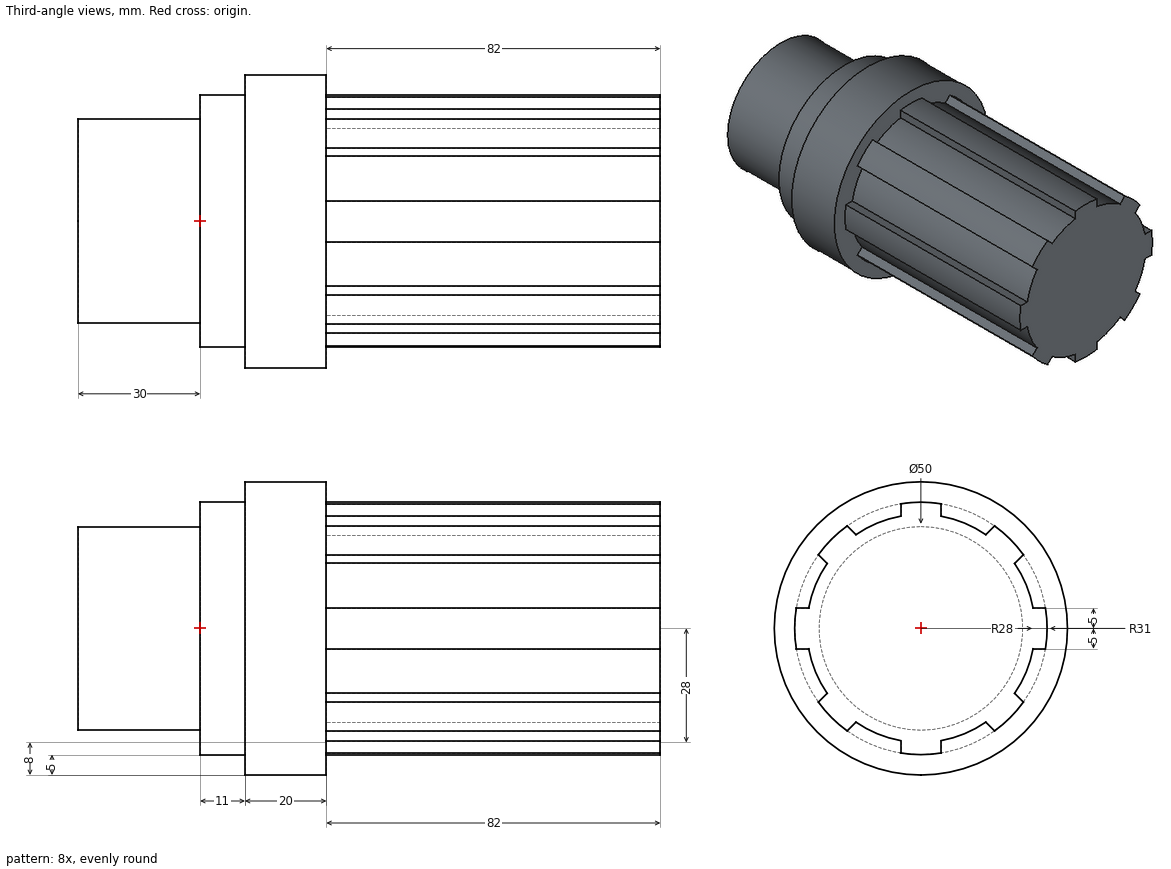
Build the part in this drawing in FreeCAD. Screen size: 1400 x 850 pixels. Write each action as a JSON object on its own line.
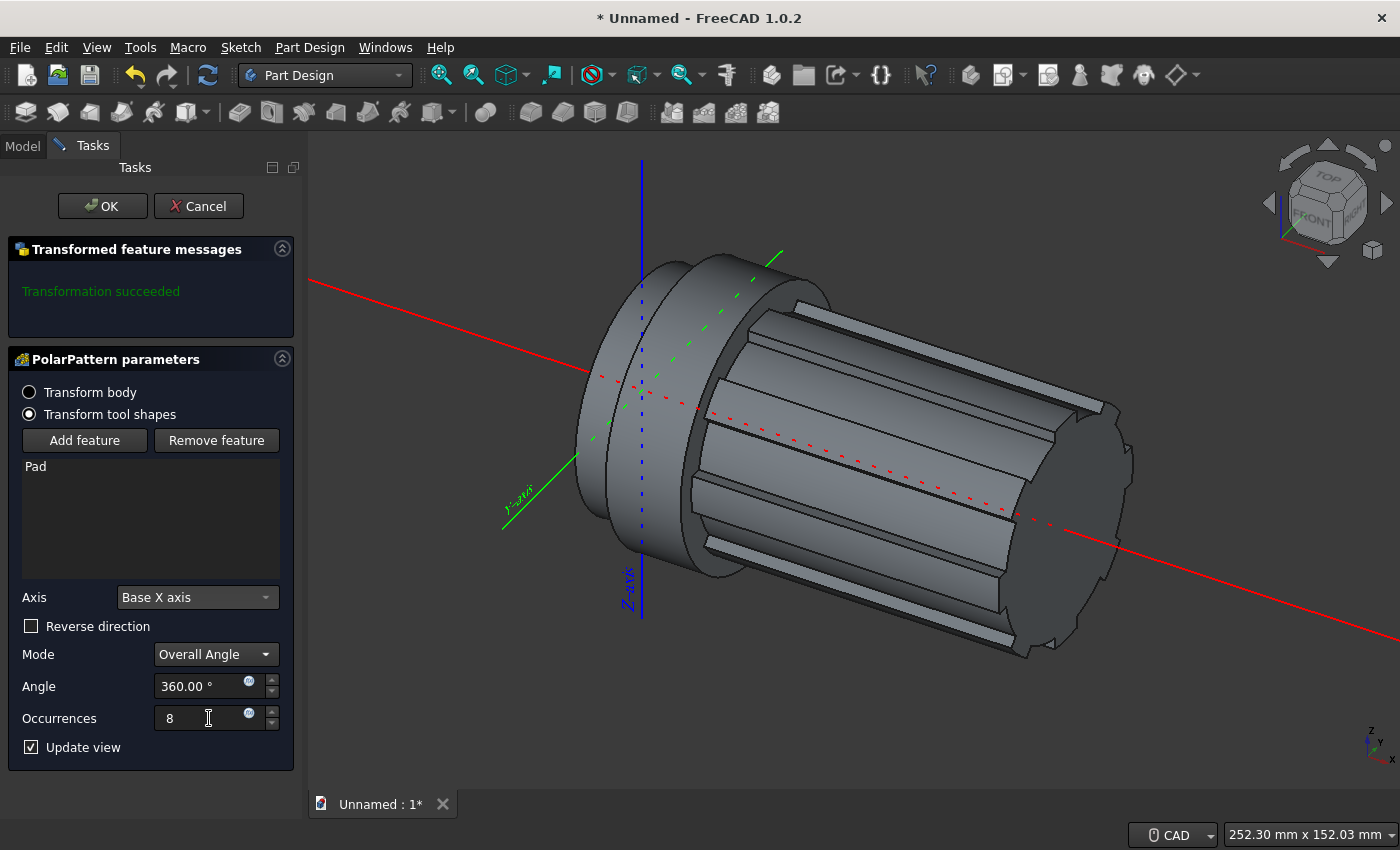
{"action": "left_click", "coordinate": [103, 206]}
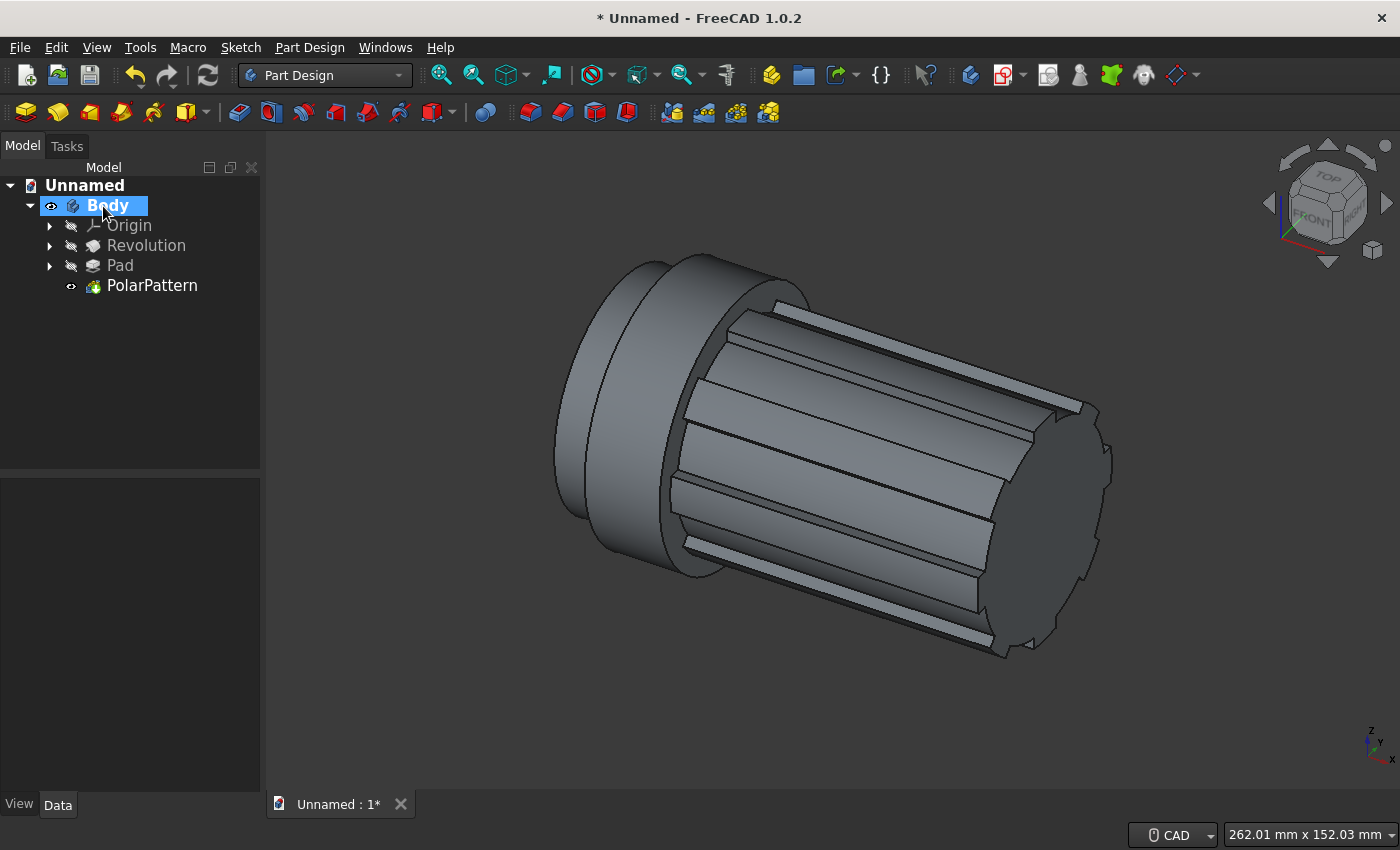
{"action": "key", "text": "6"}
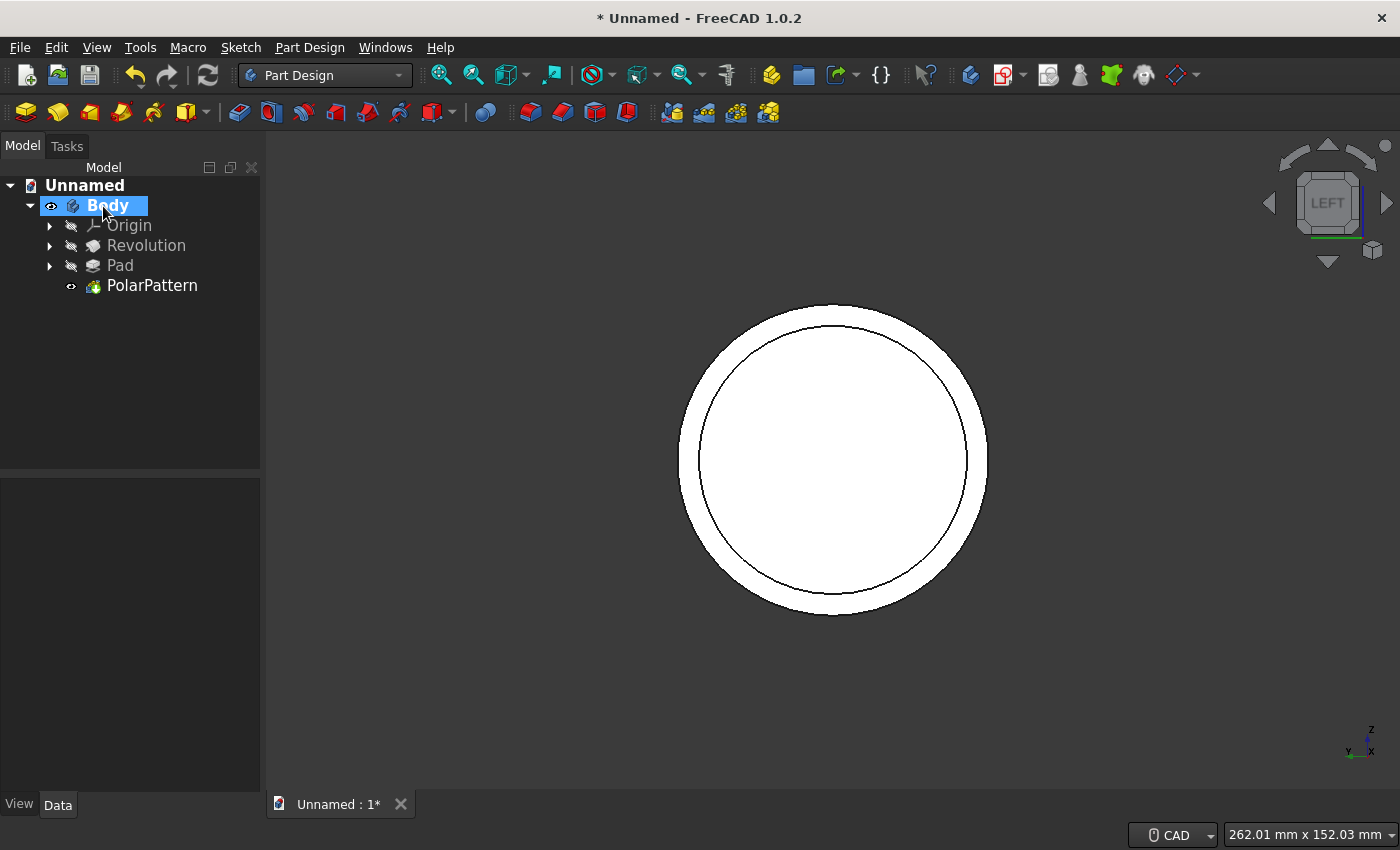
{"action": "left_click", "coordinate": [833, 459]}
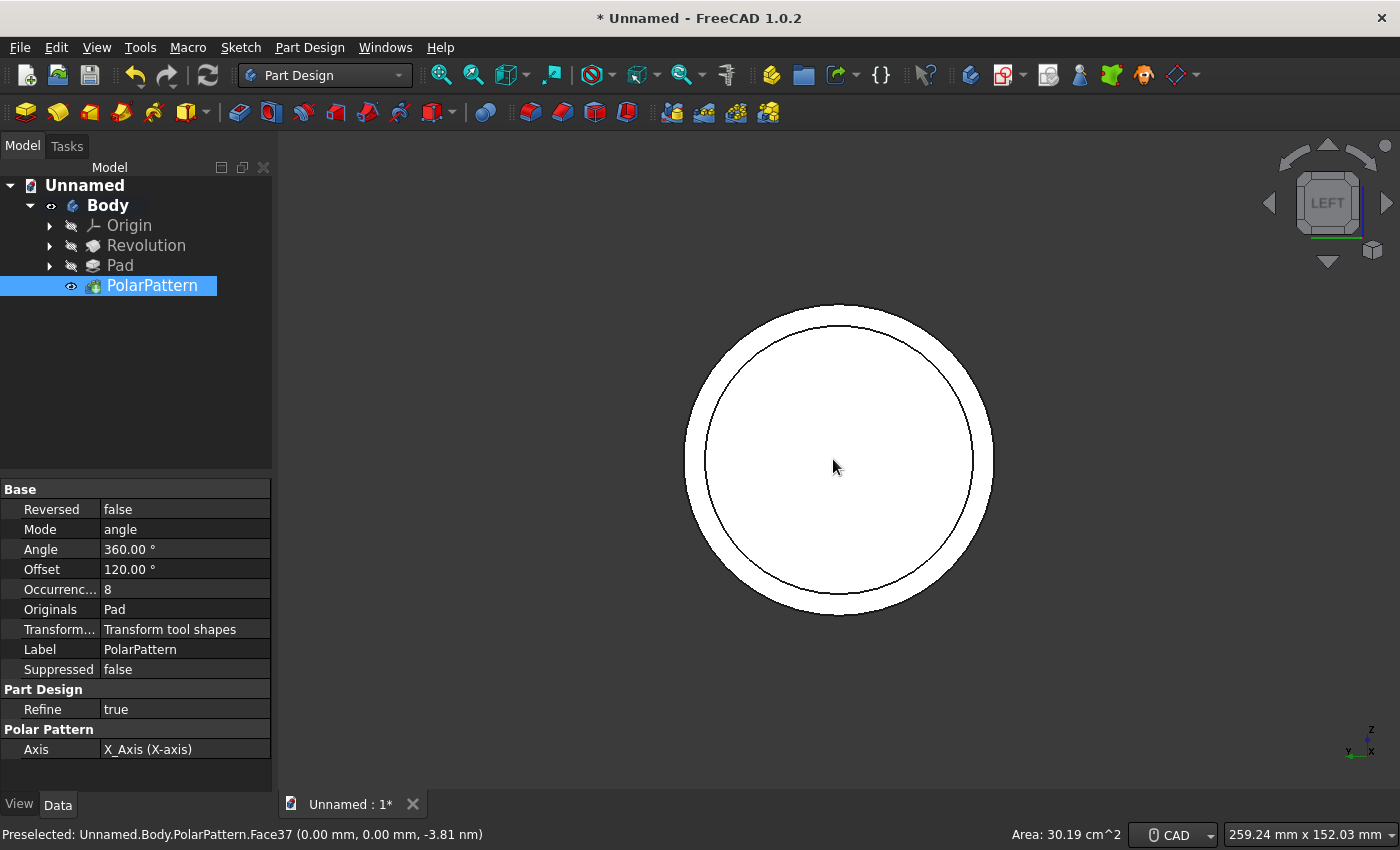
{"action": "left_click", "coordinate": [1004, 76]}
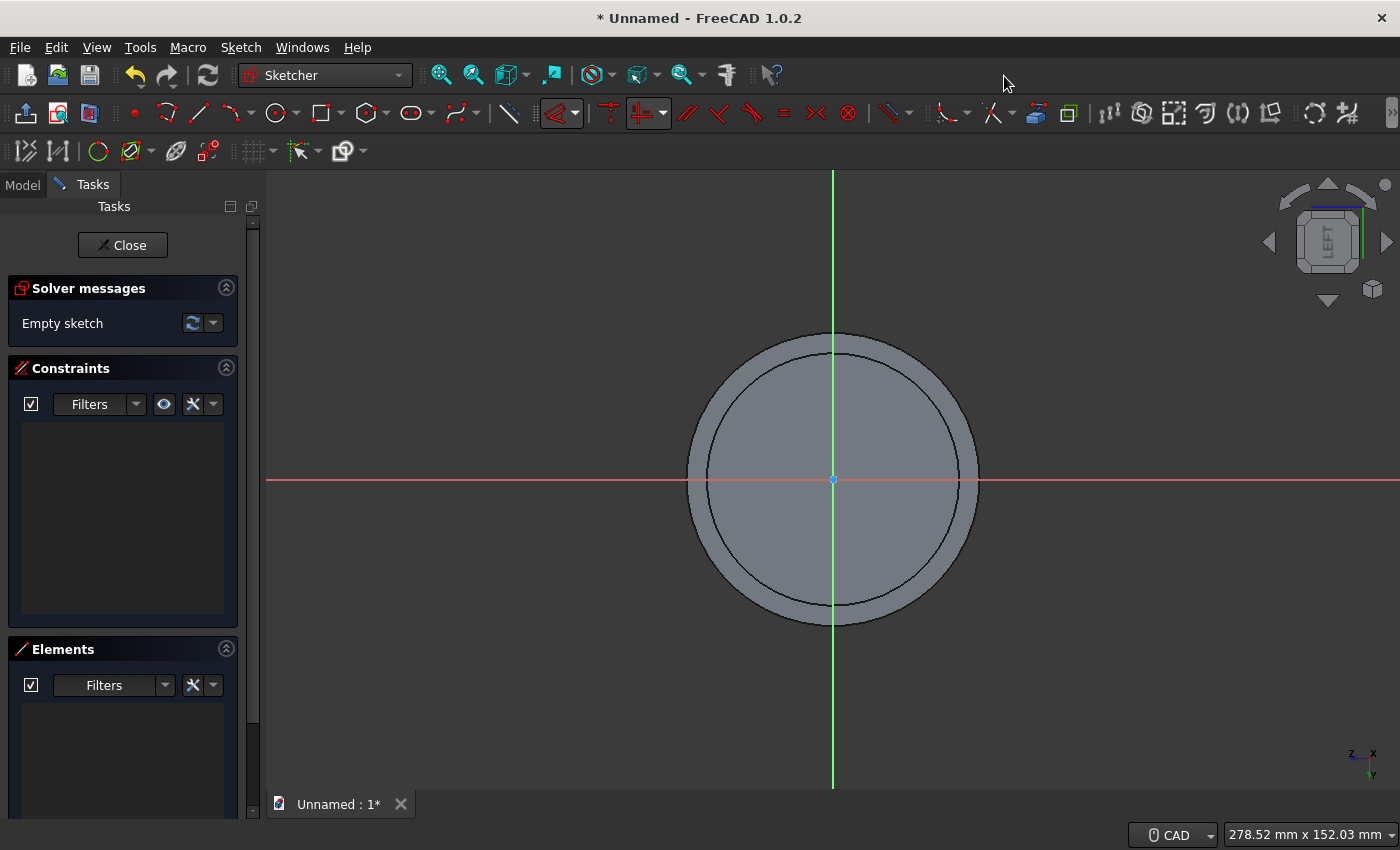
{"action": "scroll", "coordinate": [916, 480], "scroll_direction": "up", "scroll_amount": 3}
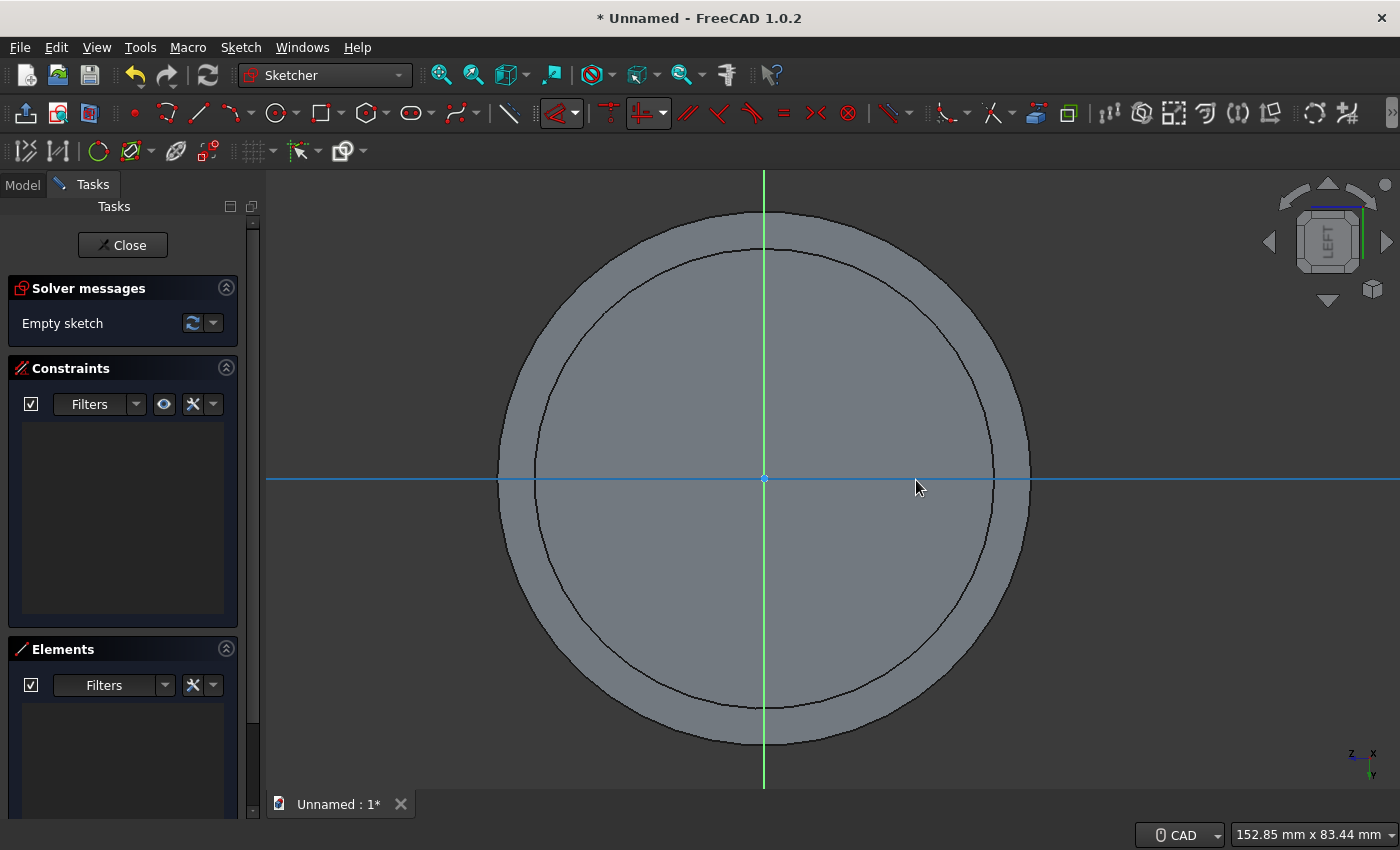
{"action": "left_click", "coordinate": [276, 114]}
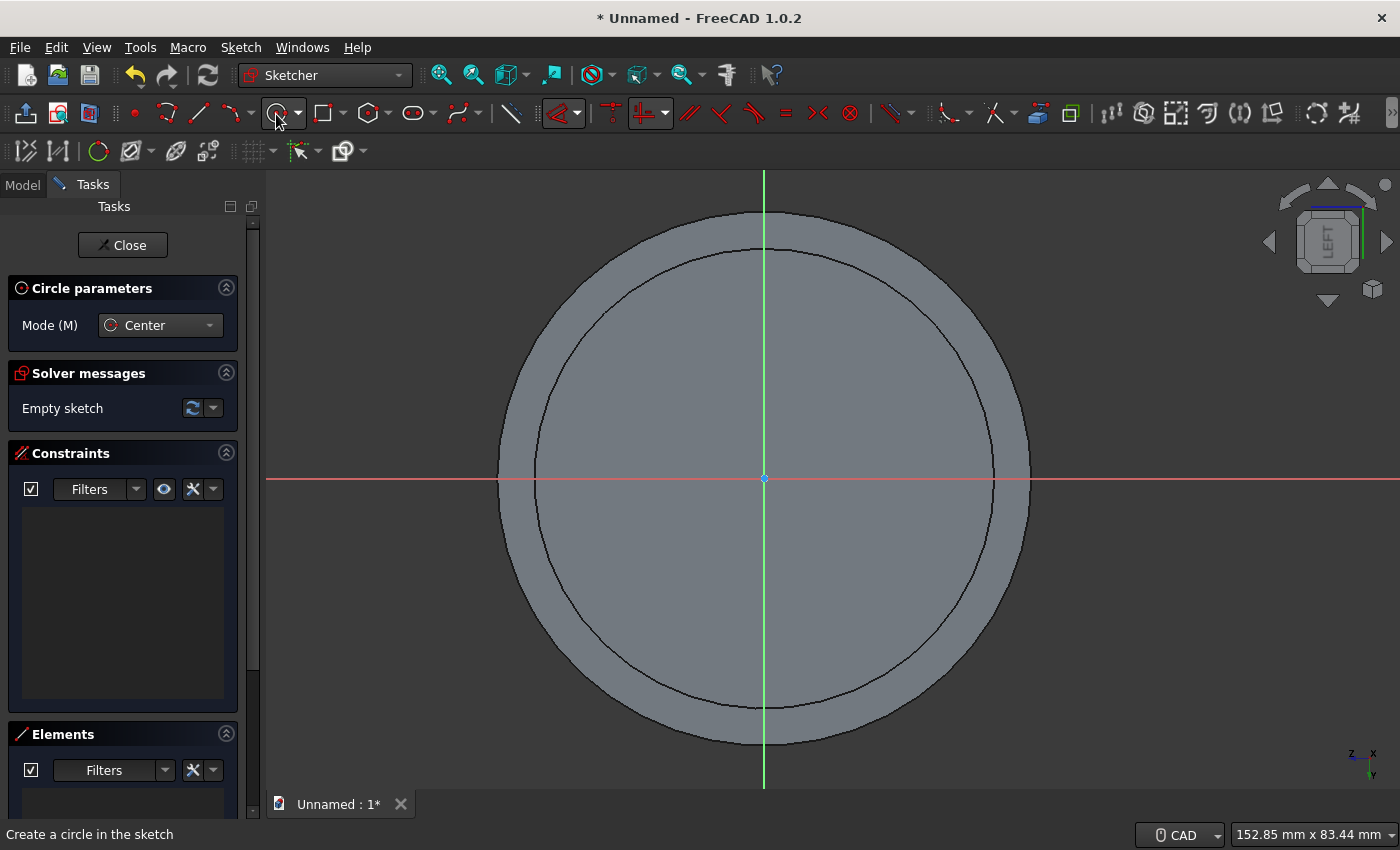
{"action": "left_click", "coordinate": [764, 479]}
{"action": "left_click", "coordinate": [895, 348]}
{"action": "key", "text": "Escape"}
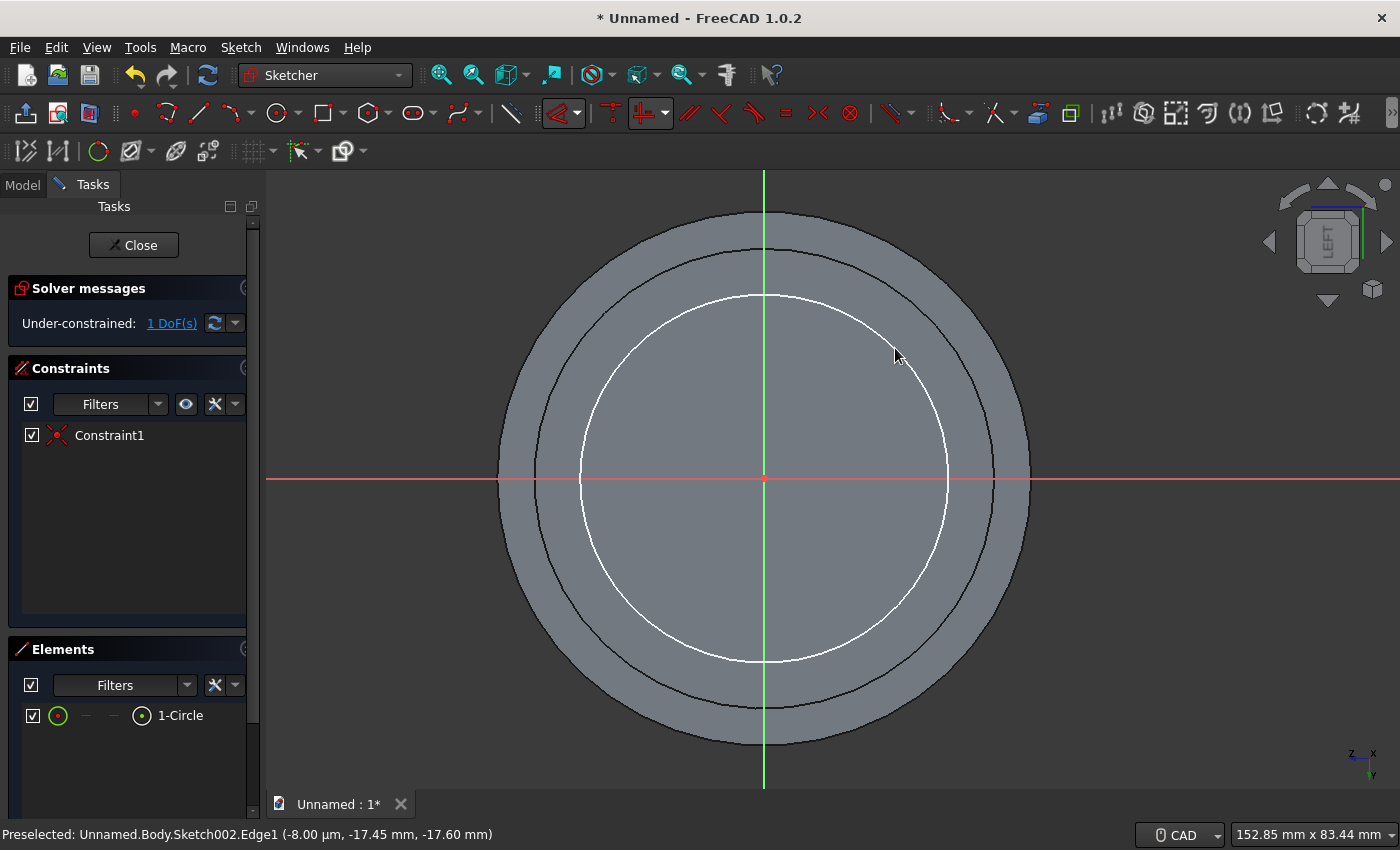
{"action": "left_click", "coordinate": [894, 348]}